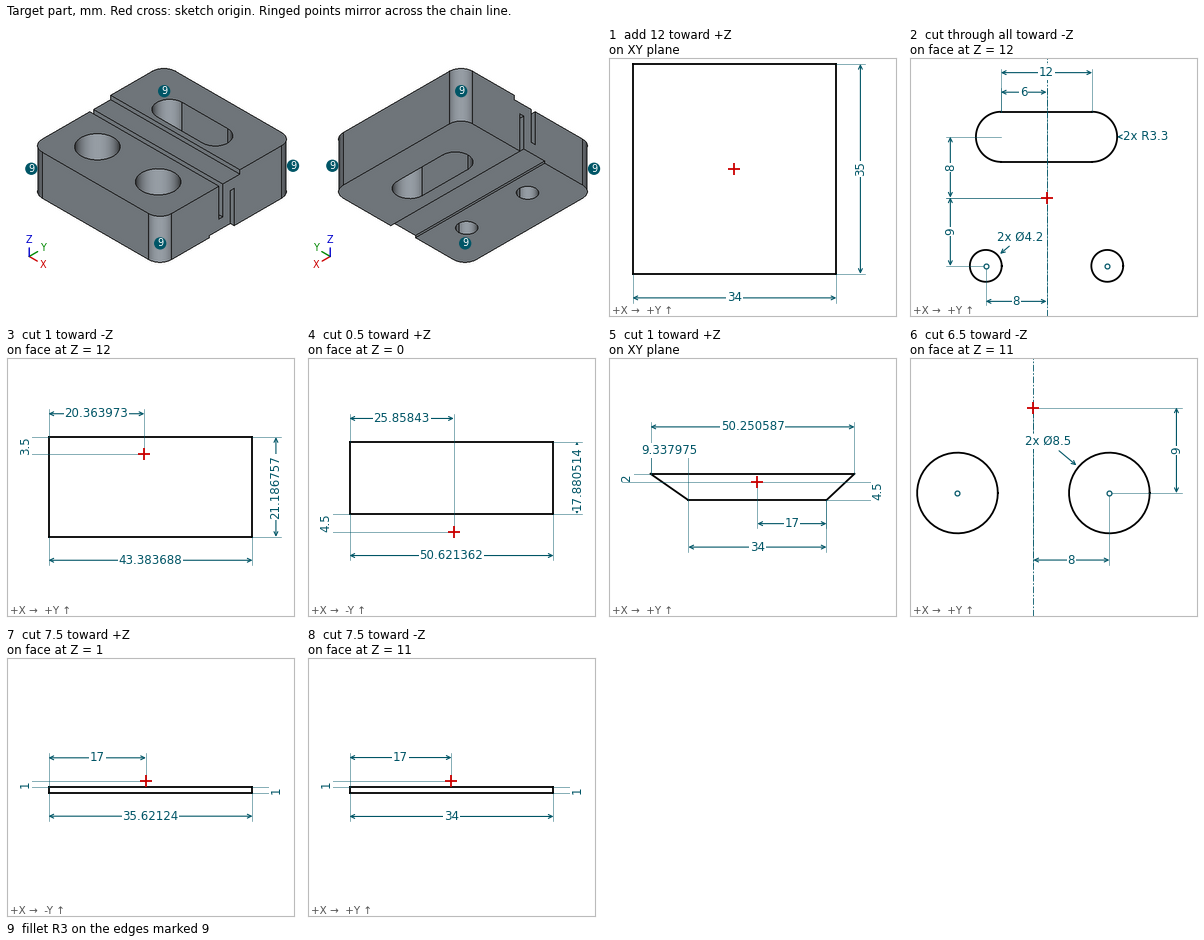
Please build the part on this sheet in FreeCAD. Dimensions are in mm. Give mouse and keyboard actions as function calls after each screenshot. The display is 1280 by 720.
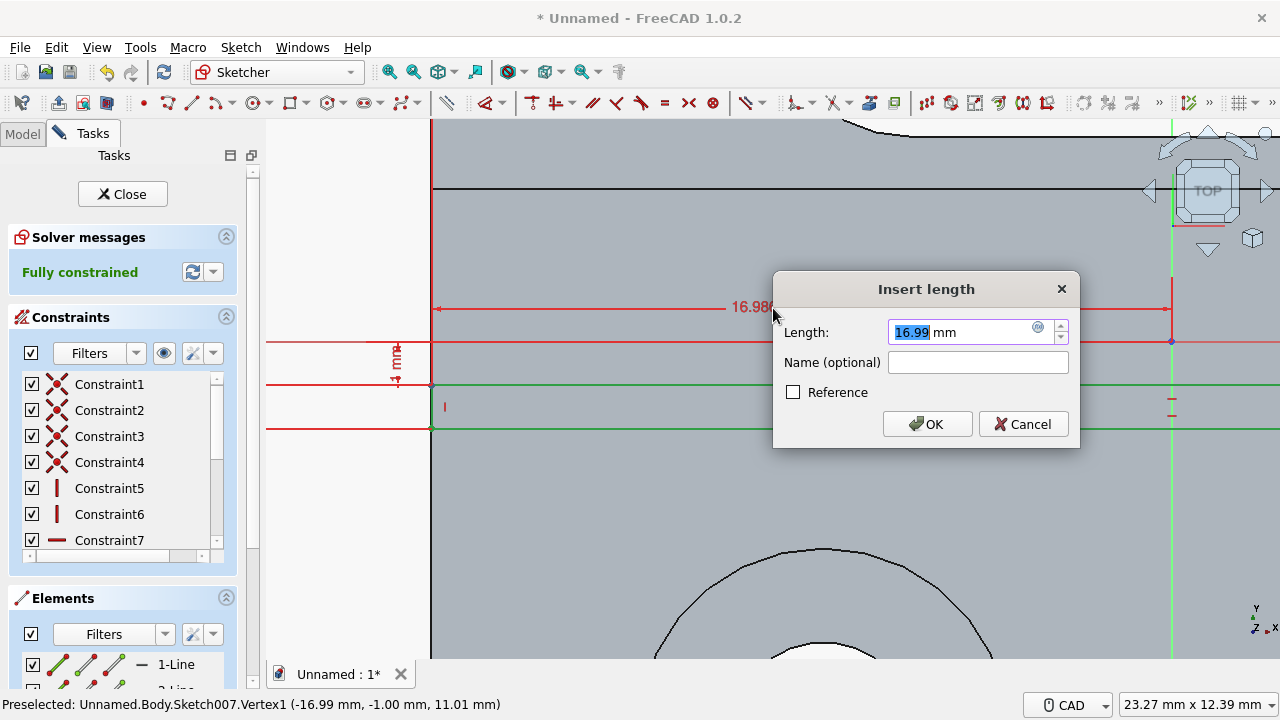
text(17)
key(Return)
key(Escape)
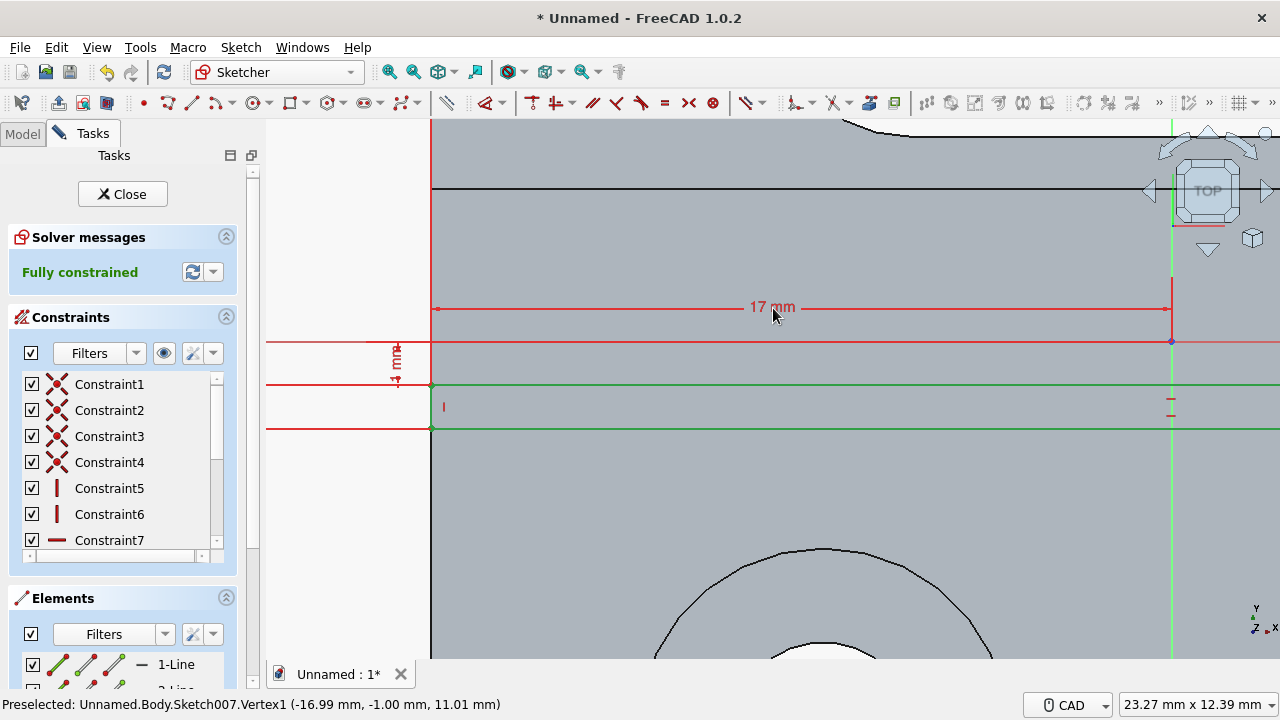
click(123, 194)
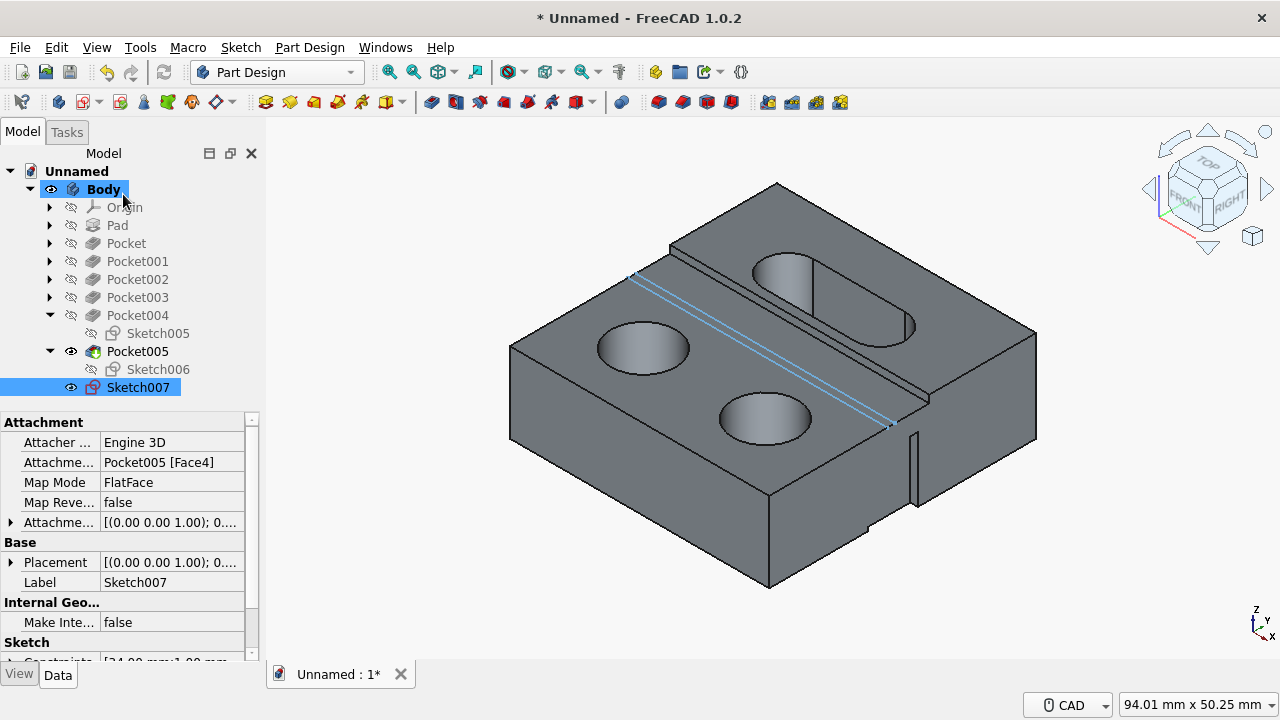
click(432, 102)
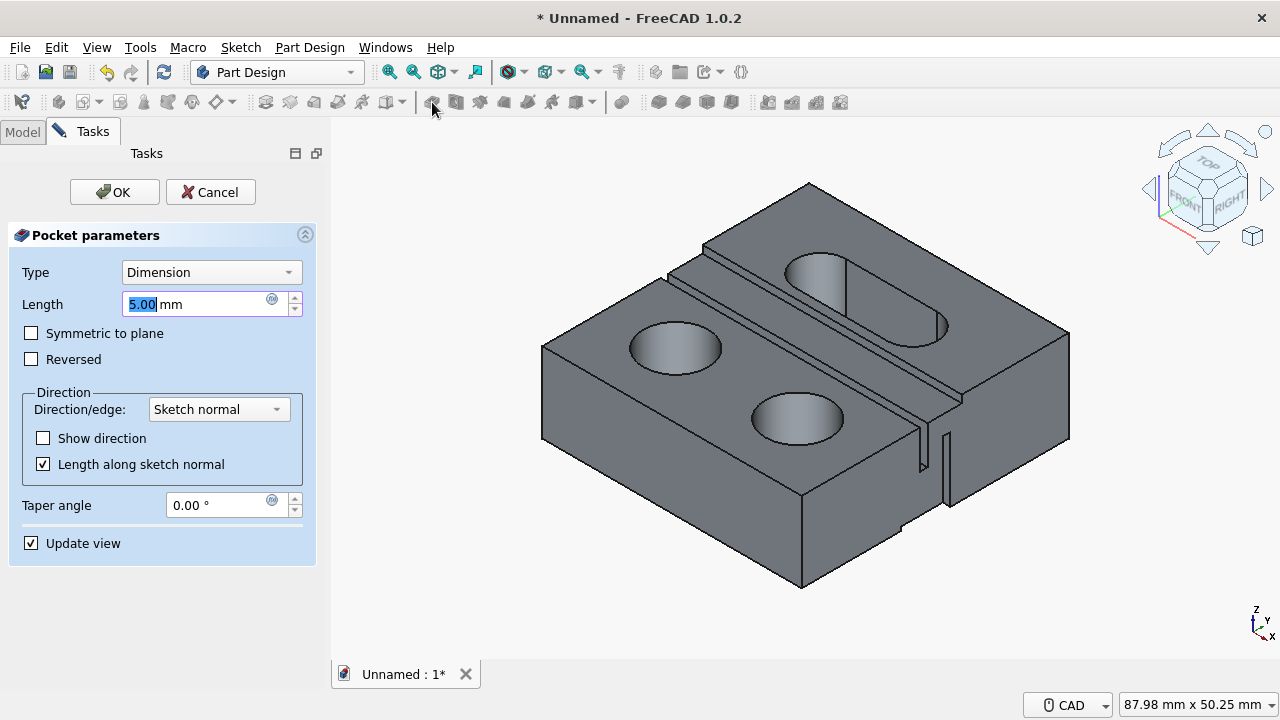
text(7.5)
key(Tab)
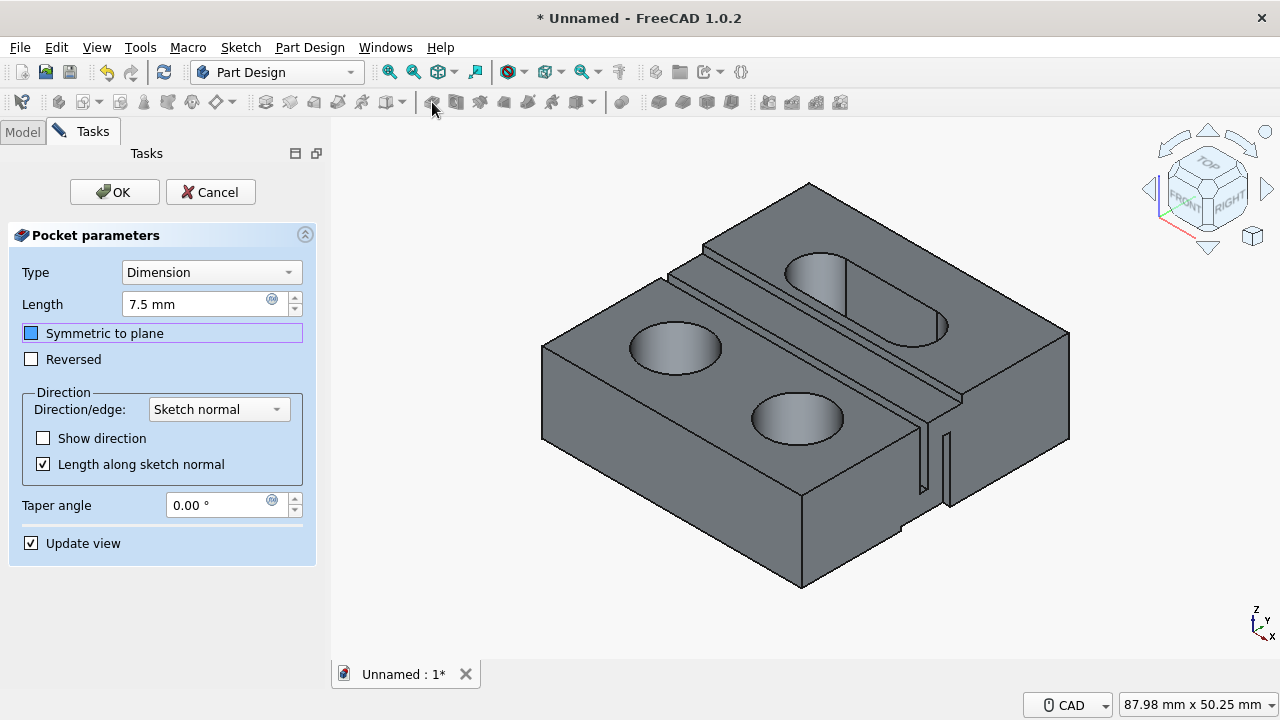
click(115, 192)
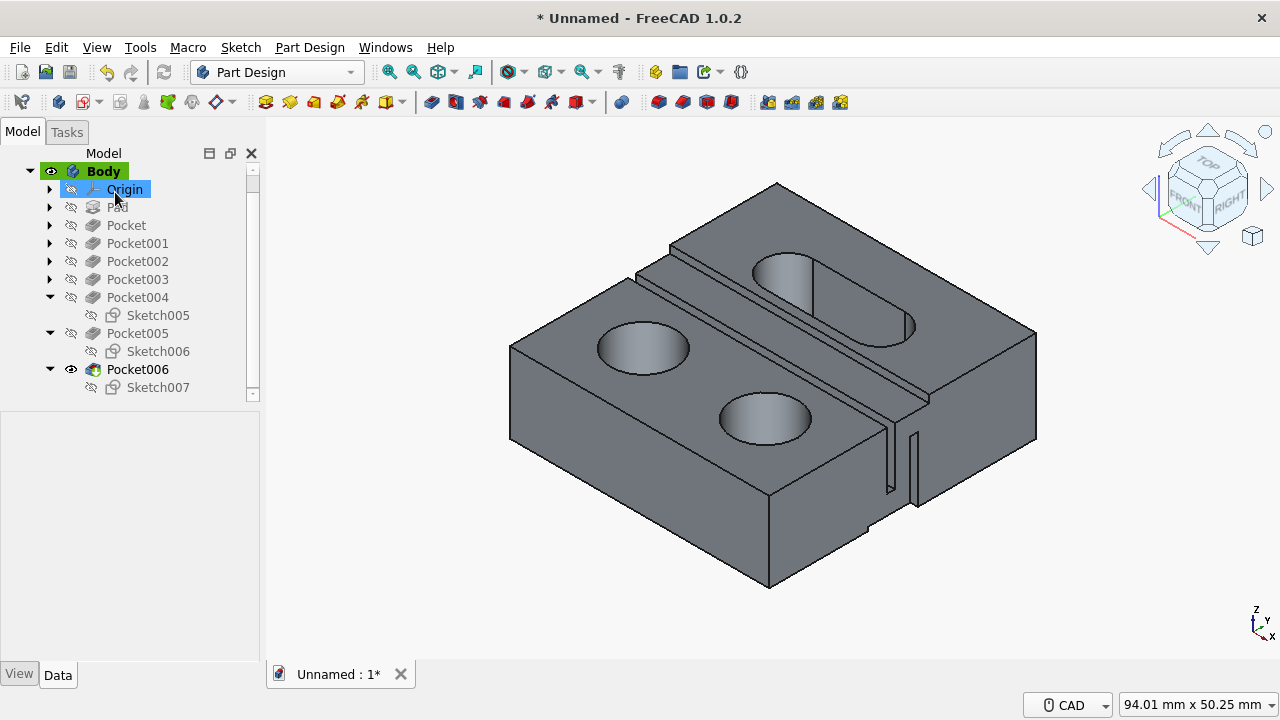
click(769, 541)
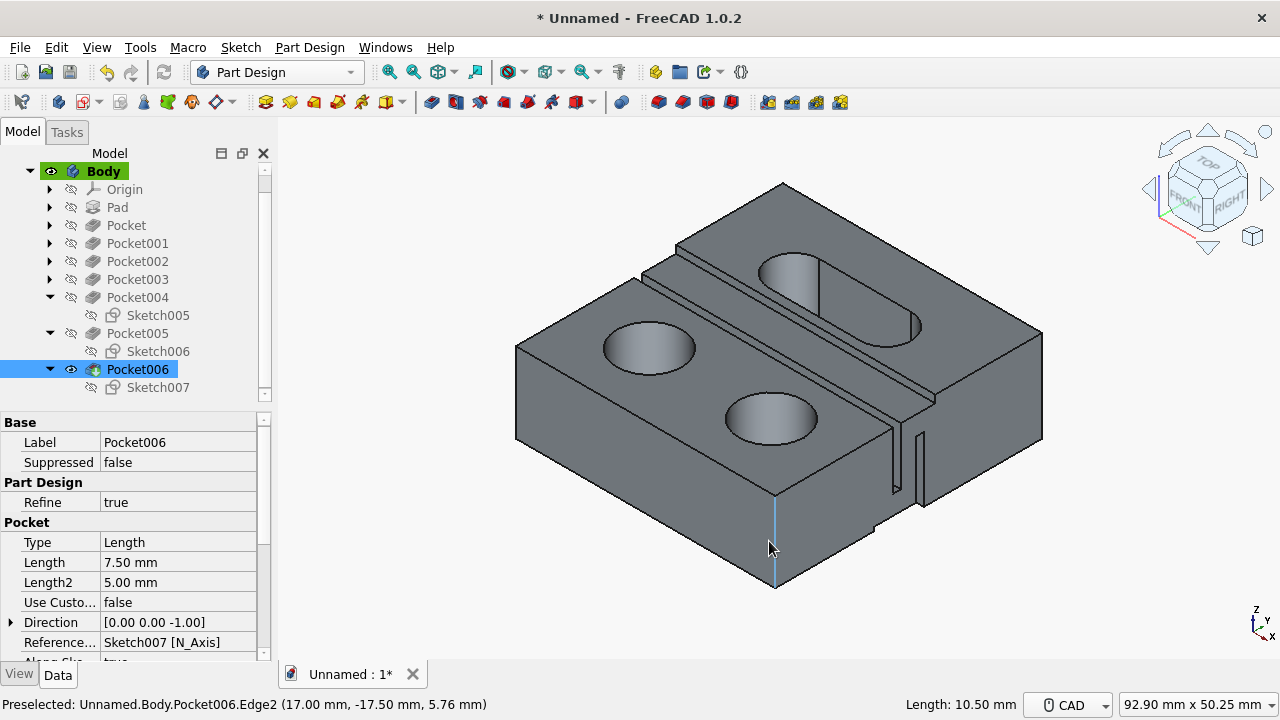
key(2)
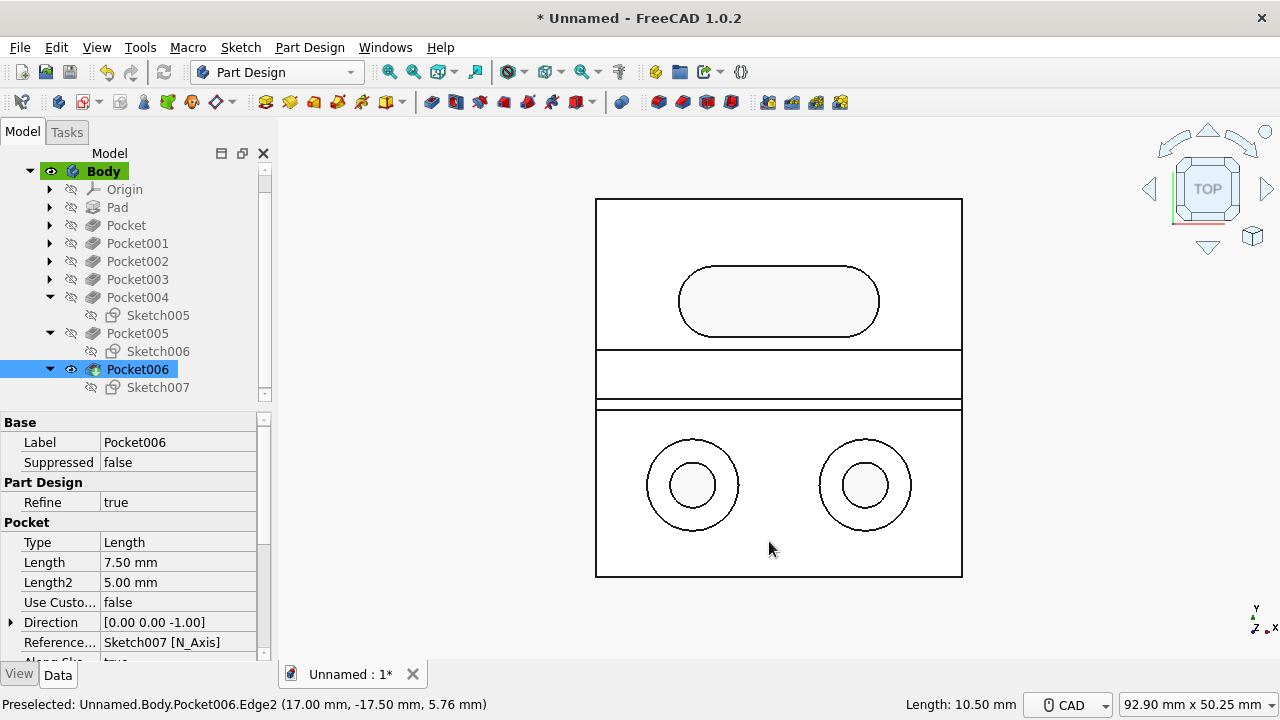
key(0)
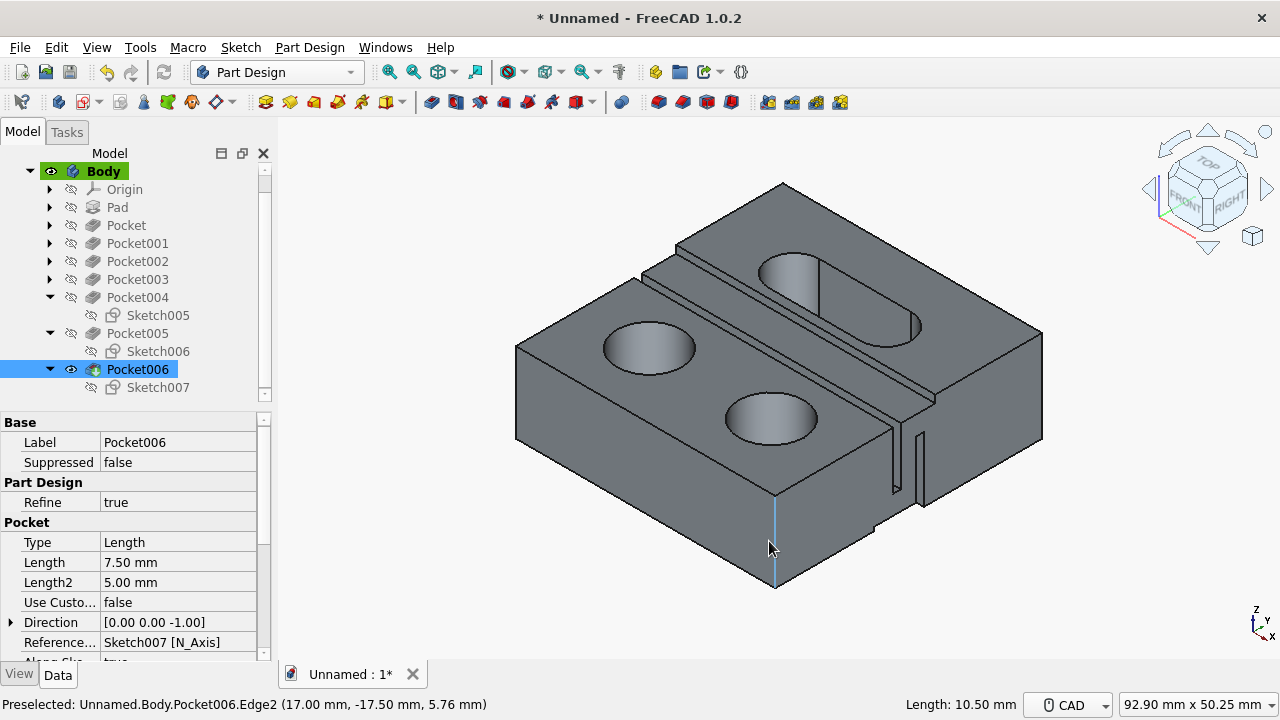
key(1)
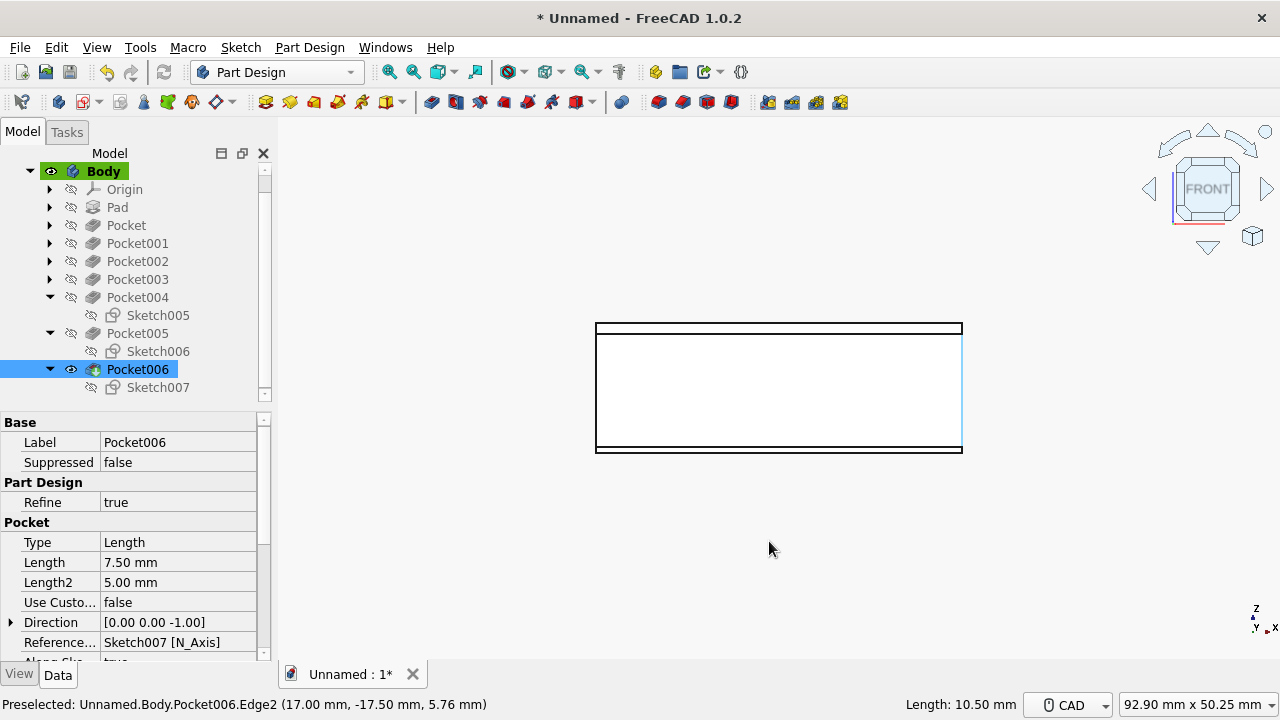
key(v)
key(f)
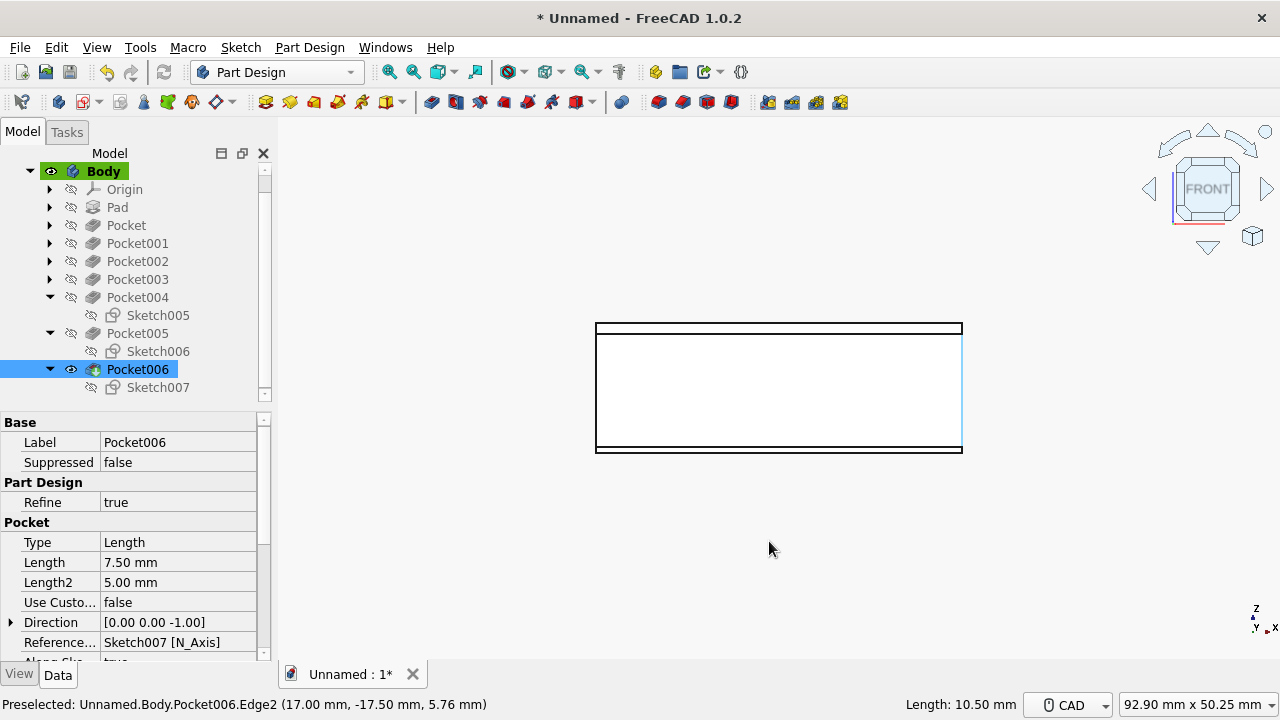
click(596, 390, ctrl)